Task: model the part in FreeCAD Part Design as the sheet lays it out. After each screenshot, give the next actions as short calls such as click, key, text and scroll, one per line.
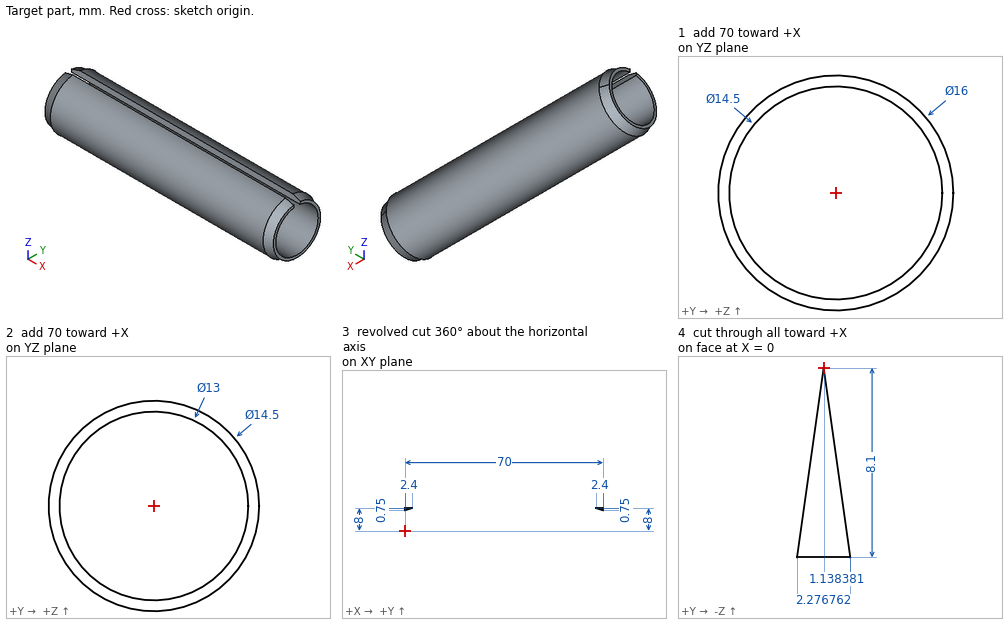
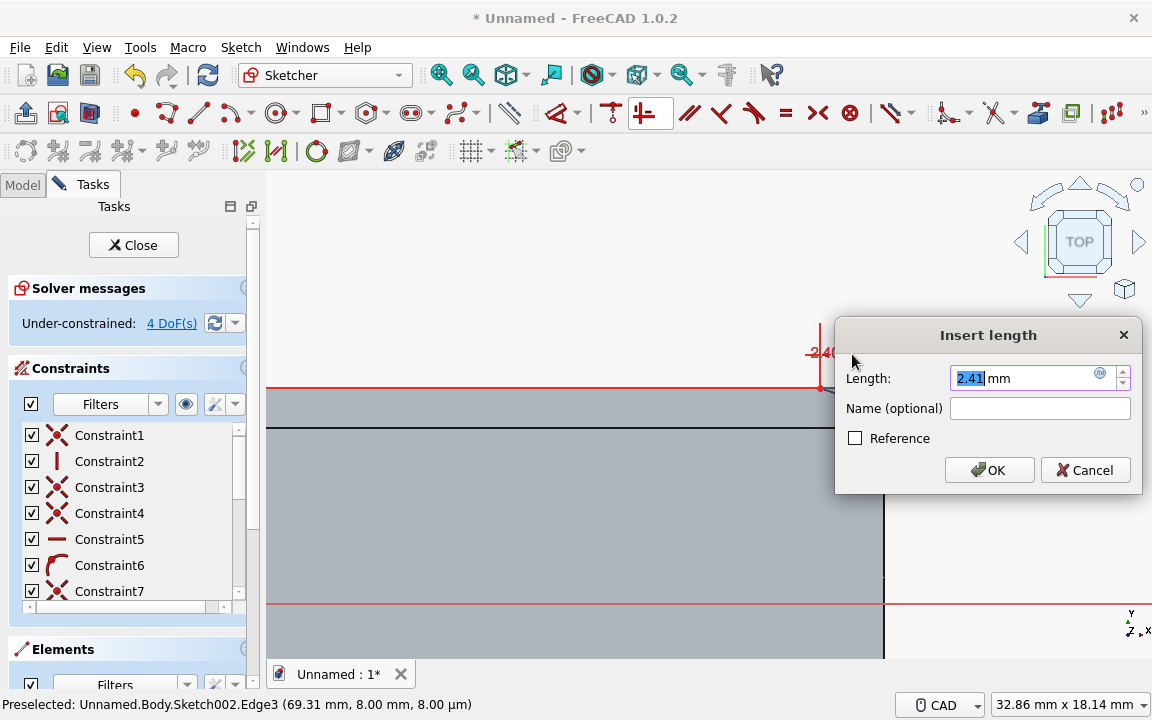
text(2.4)
key(Return)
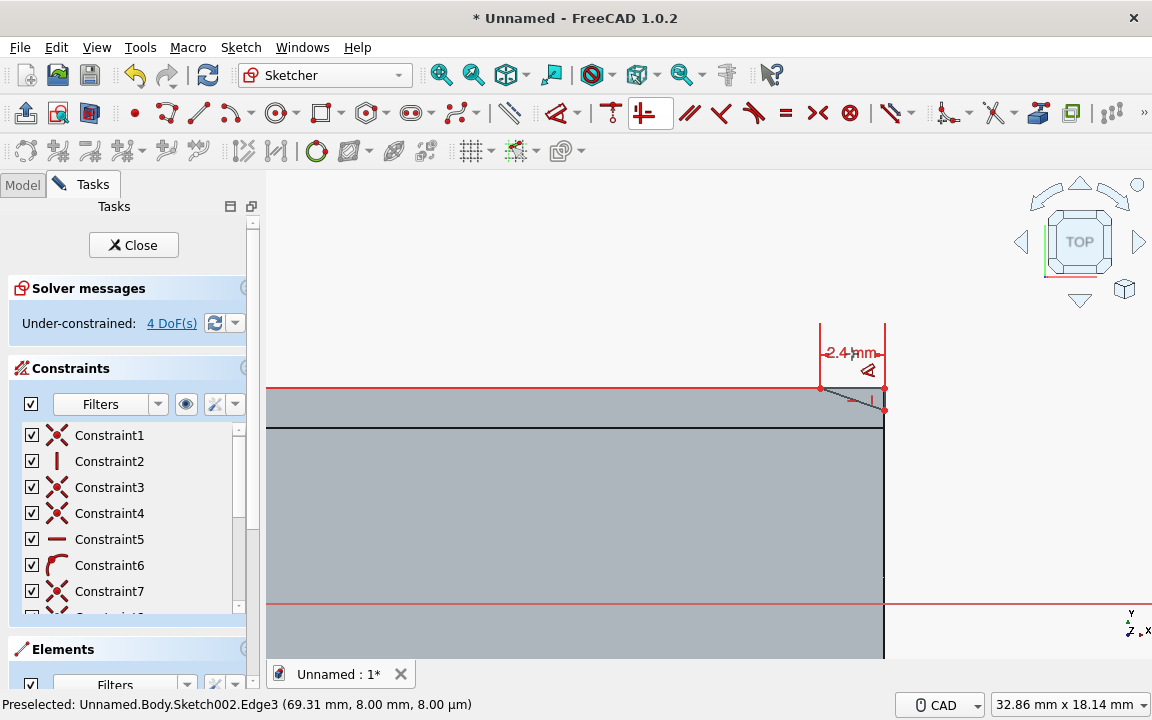
scroll(870, 388, down, 7)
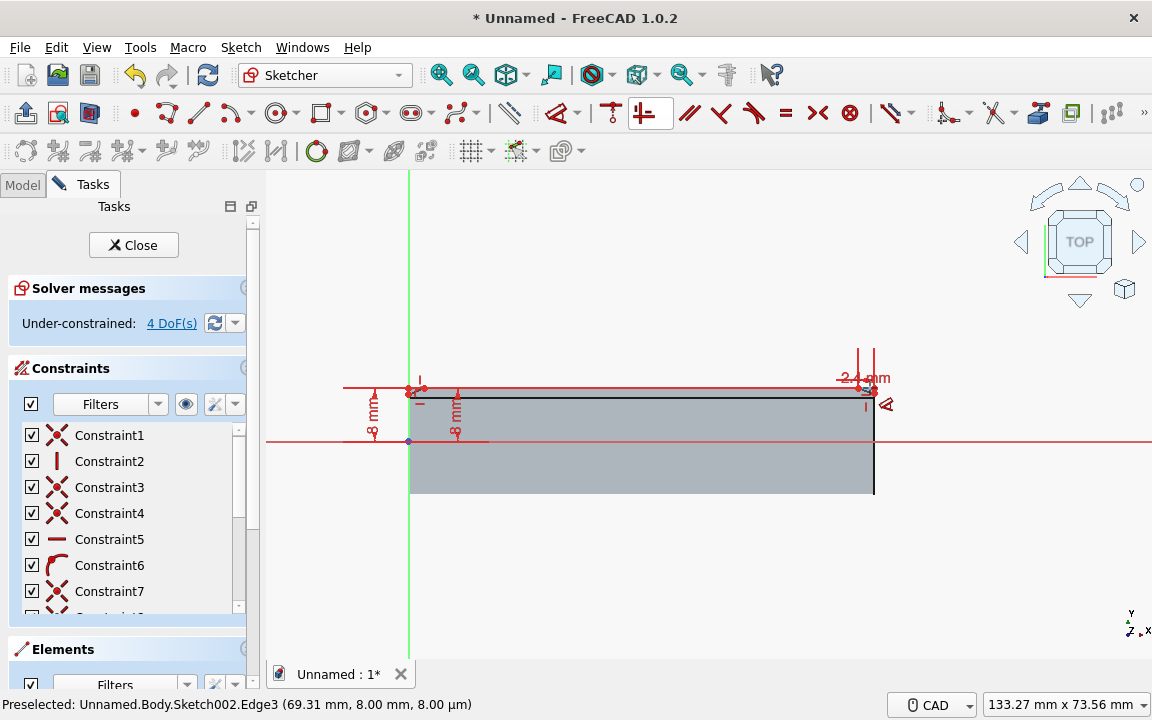
scroll(413, 388, up, 7)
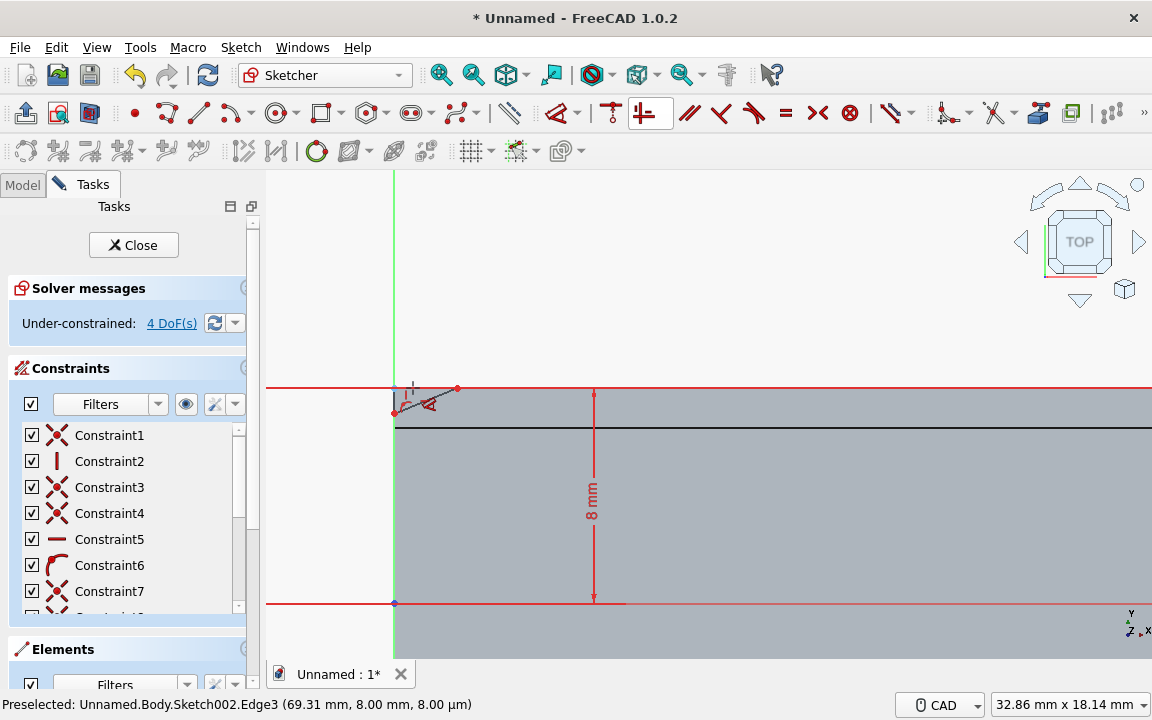
click(413, 388)
click(426, 354)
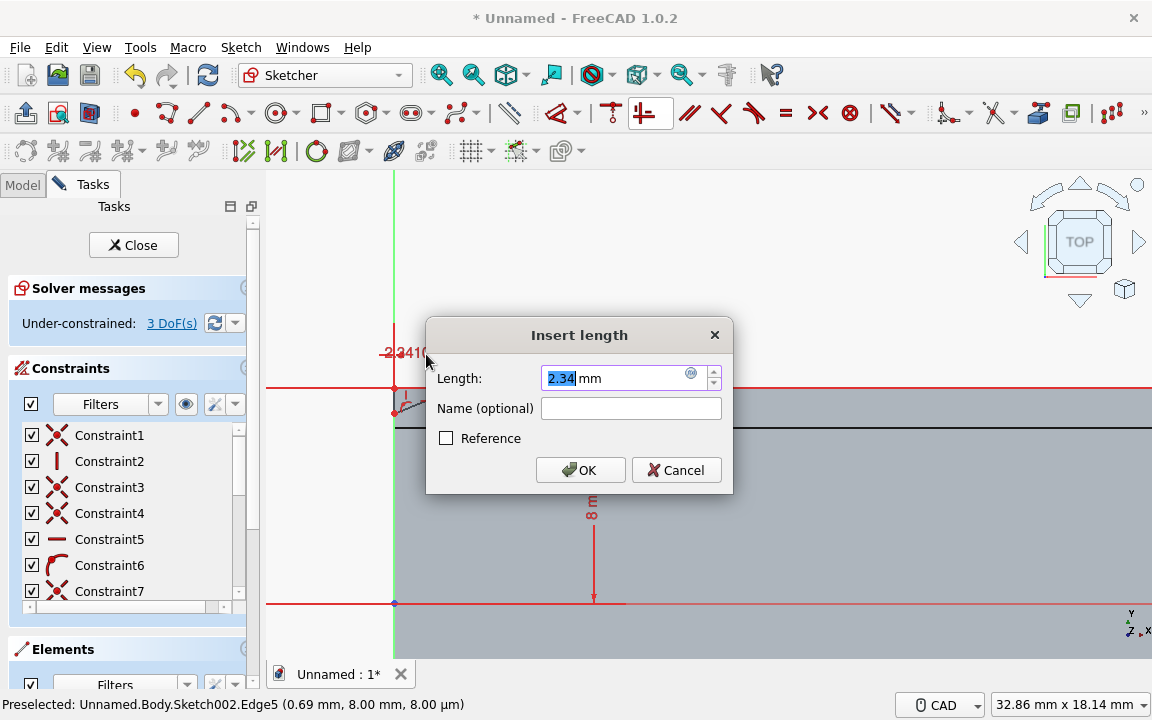
text(2.4)
key(Return)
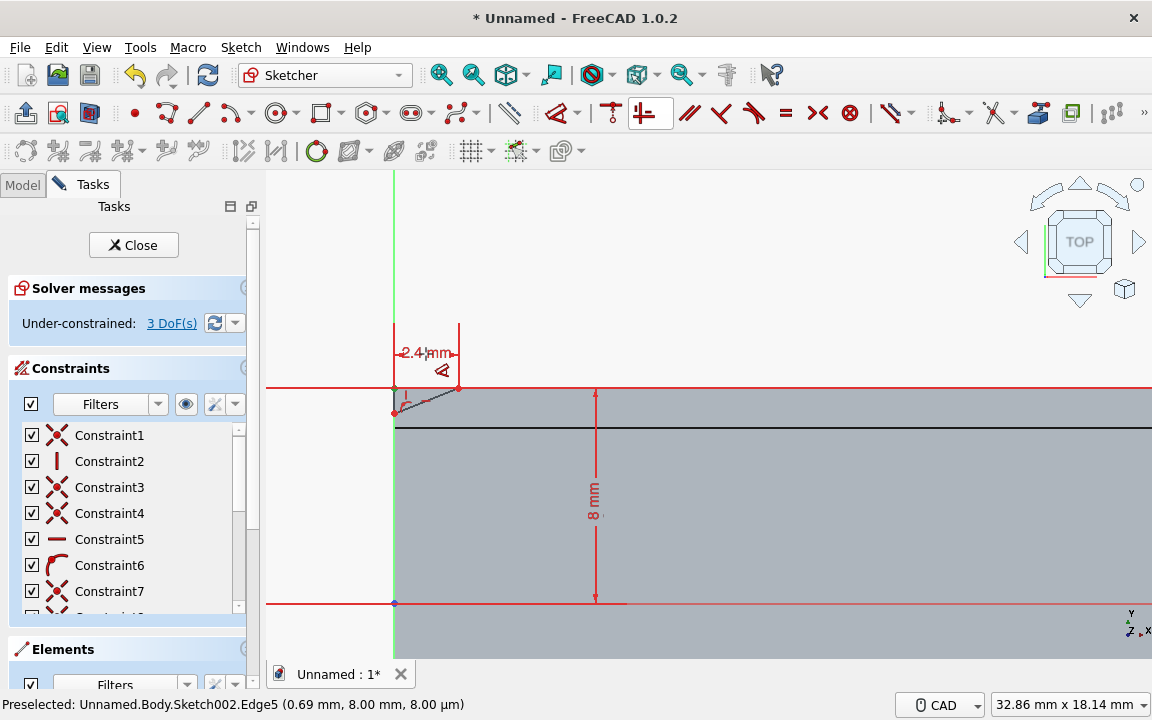
scroll(412, 388, down, 7)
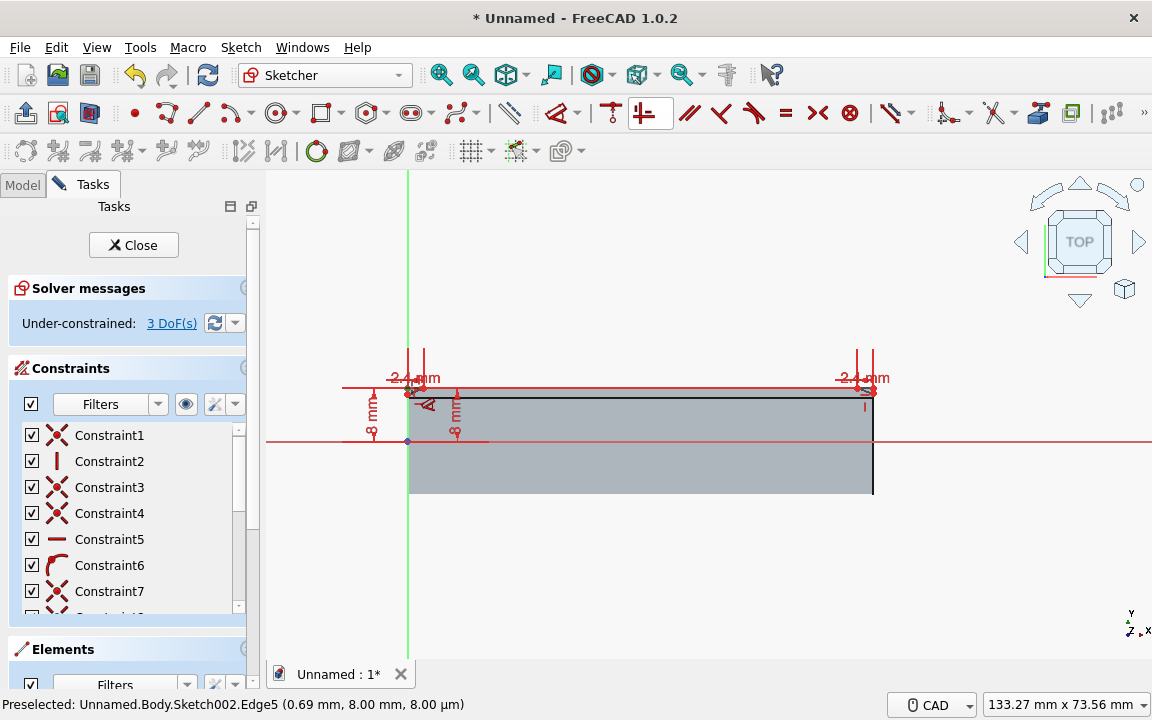
scroll(873, 394, up, 4)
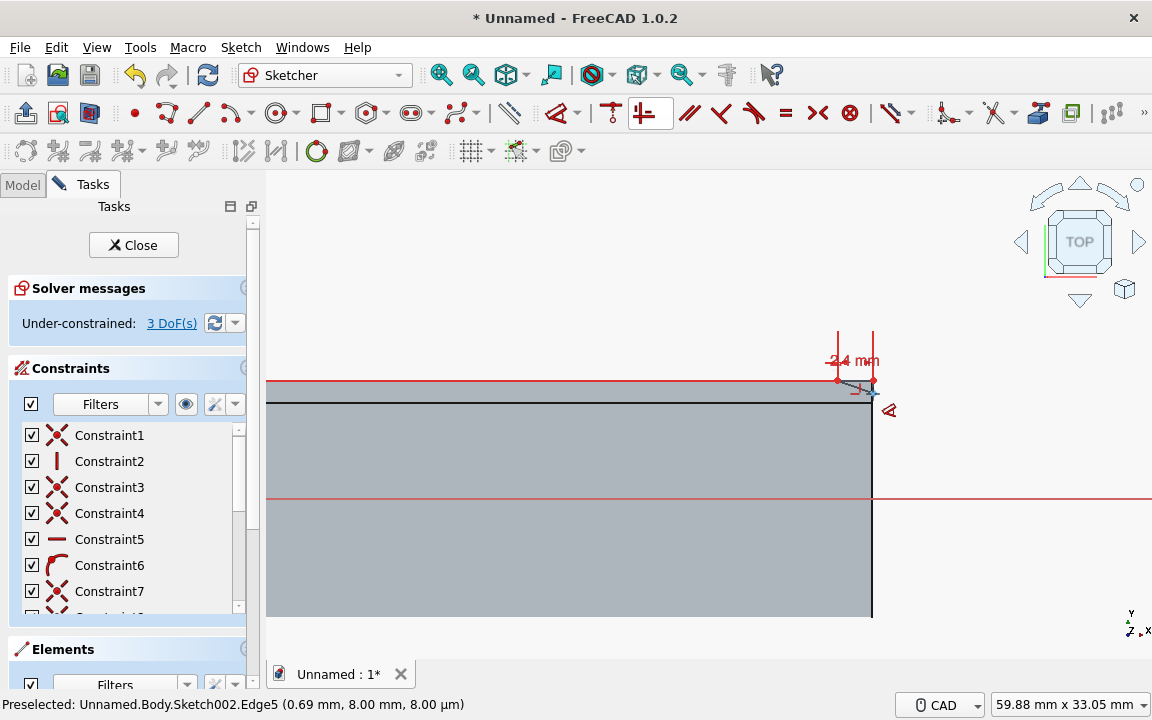
click(873, 393)
click(584, 533)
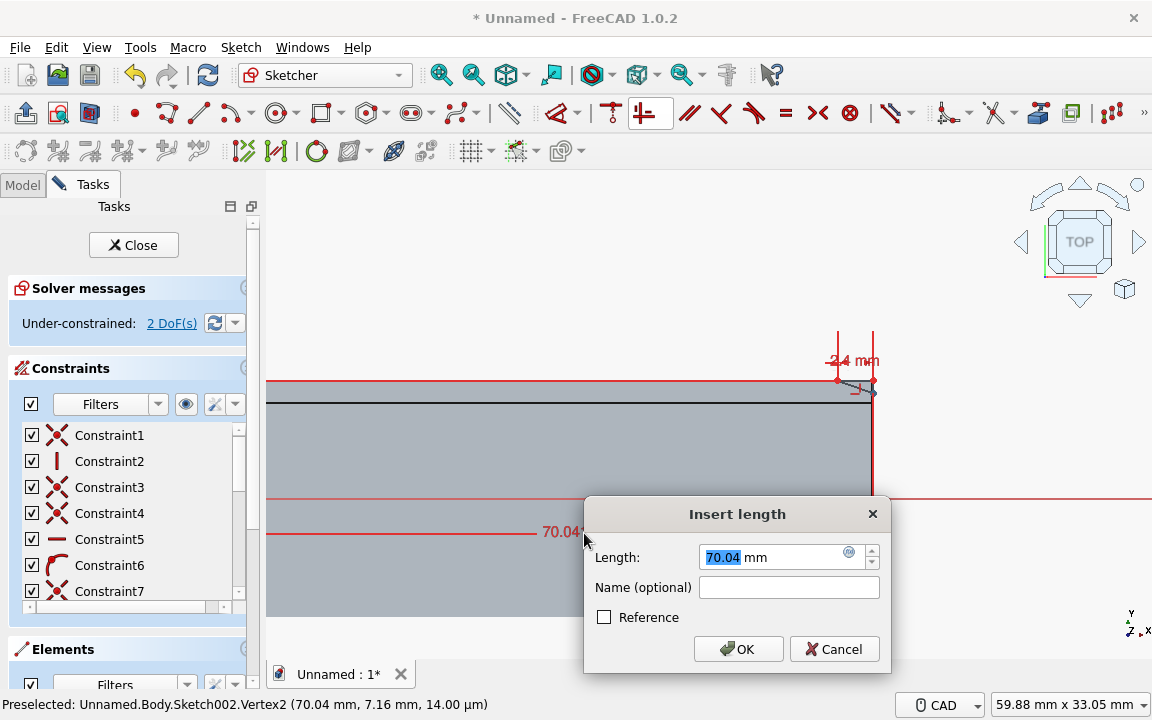
text(70)
key(Return)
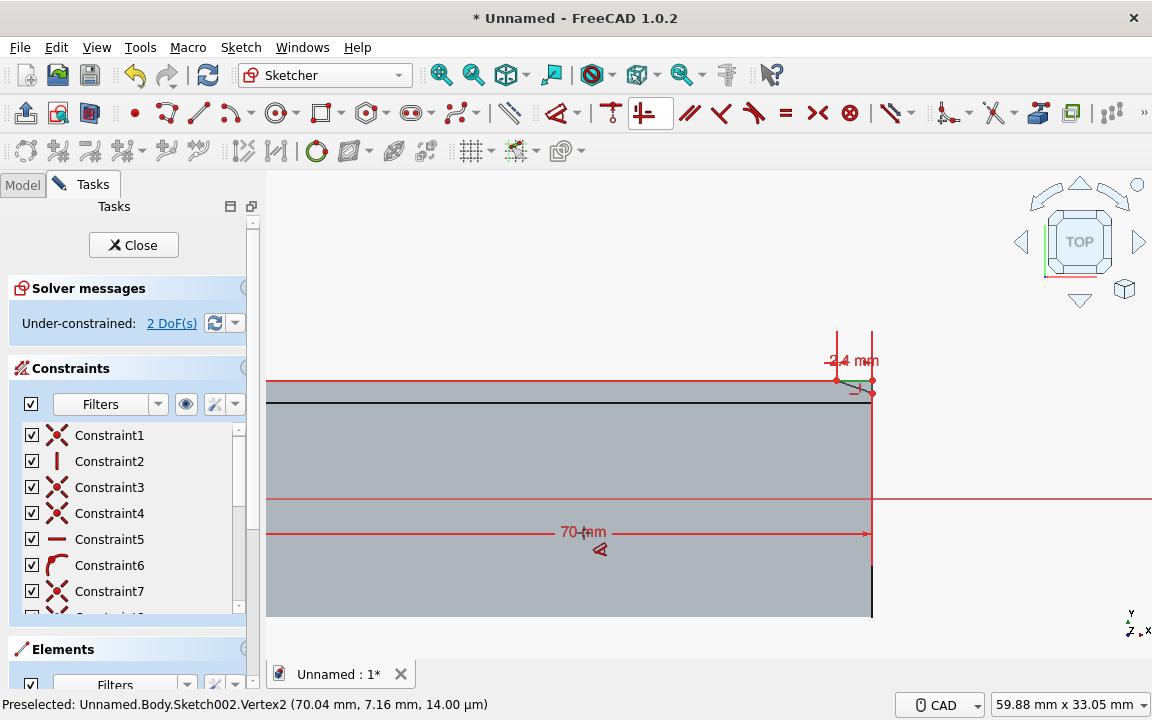
scroll(872, 387, up, 7)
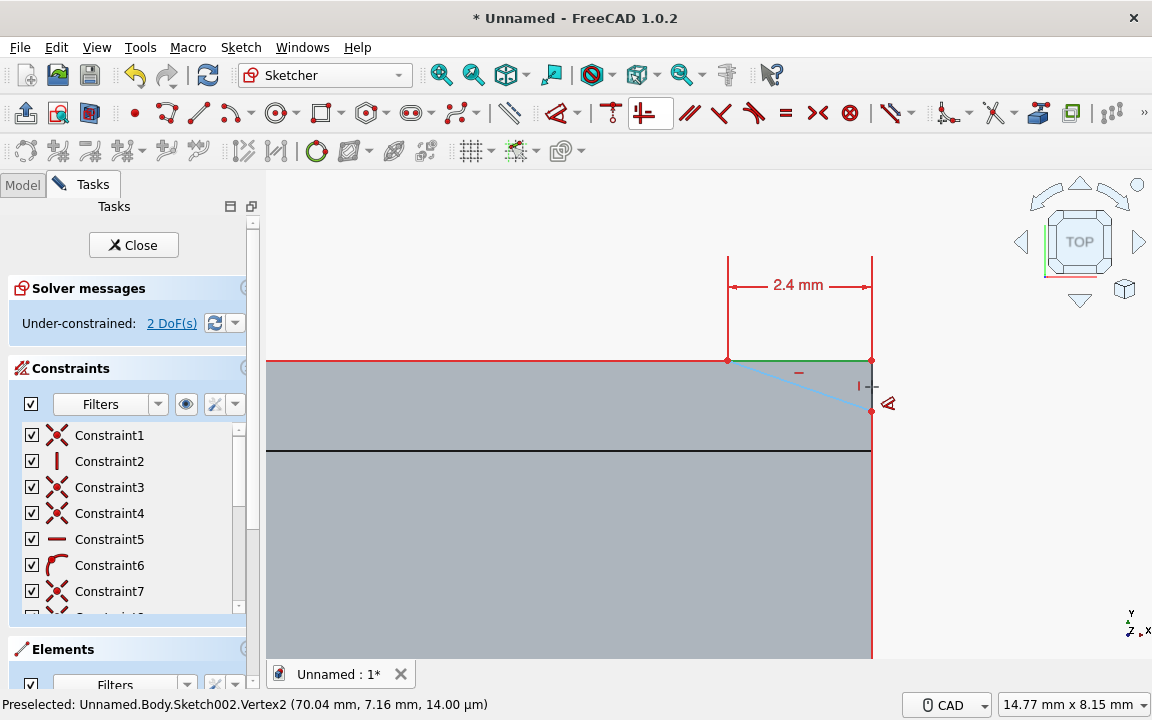
click(872, 386)
click(906, 386)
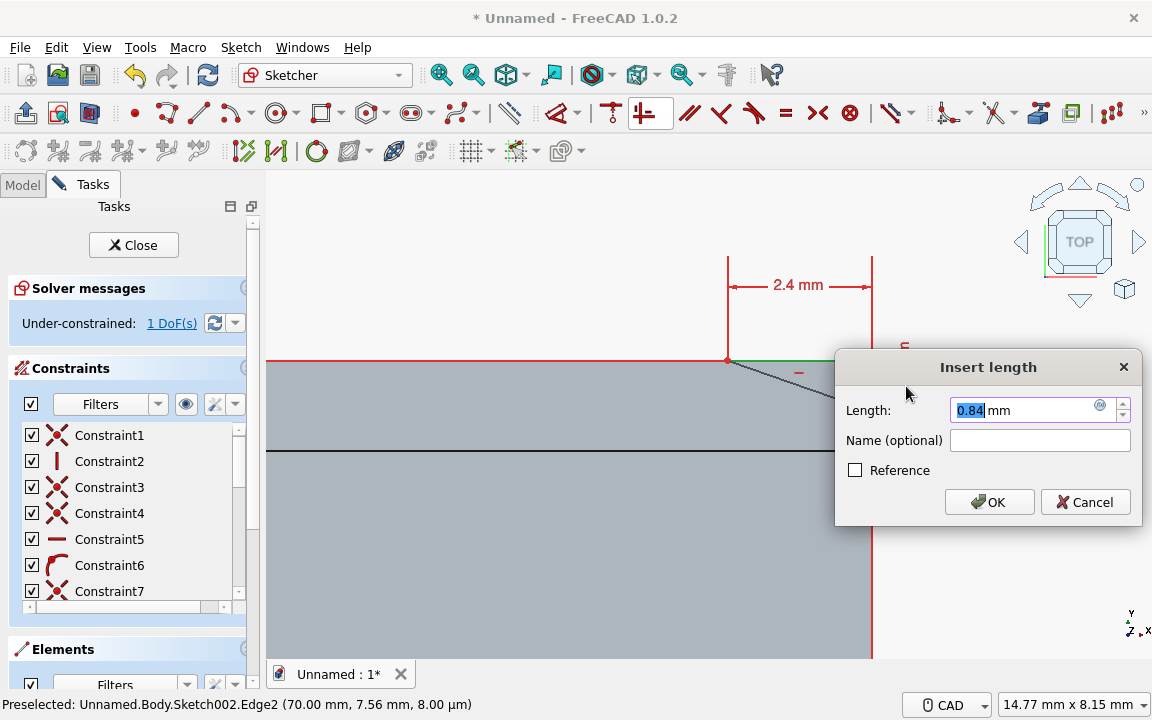
text(0.75)
key(Return)